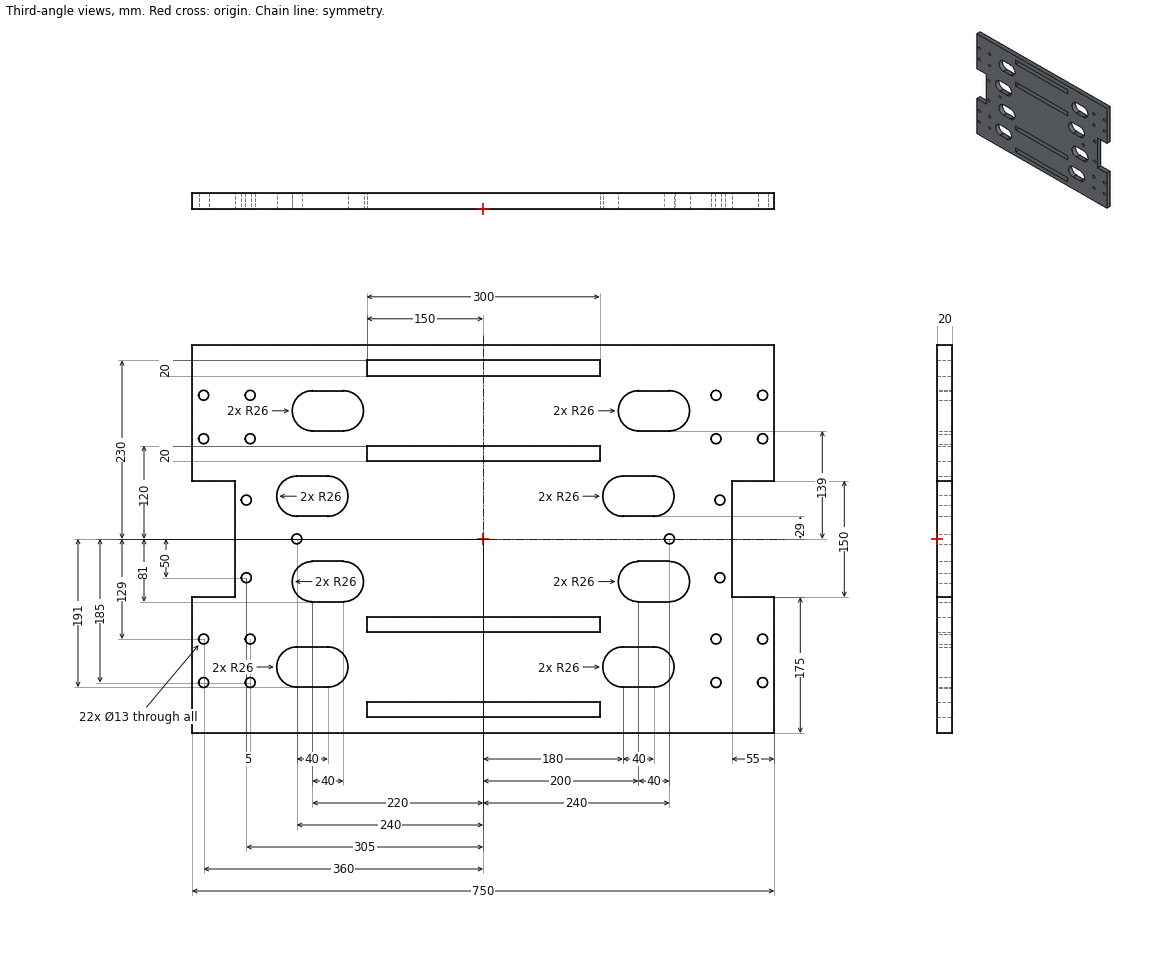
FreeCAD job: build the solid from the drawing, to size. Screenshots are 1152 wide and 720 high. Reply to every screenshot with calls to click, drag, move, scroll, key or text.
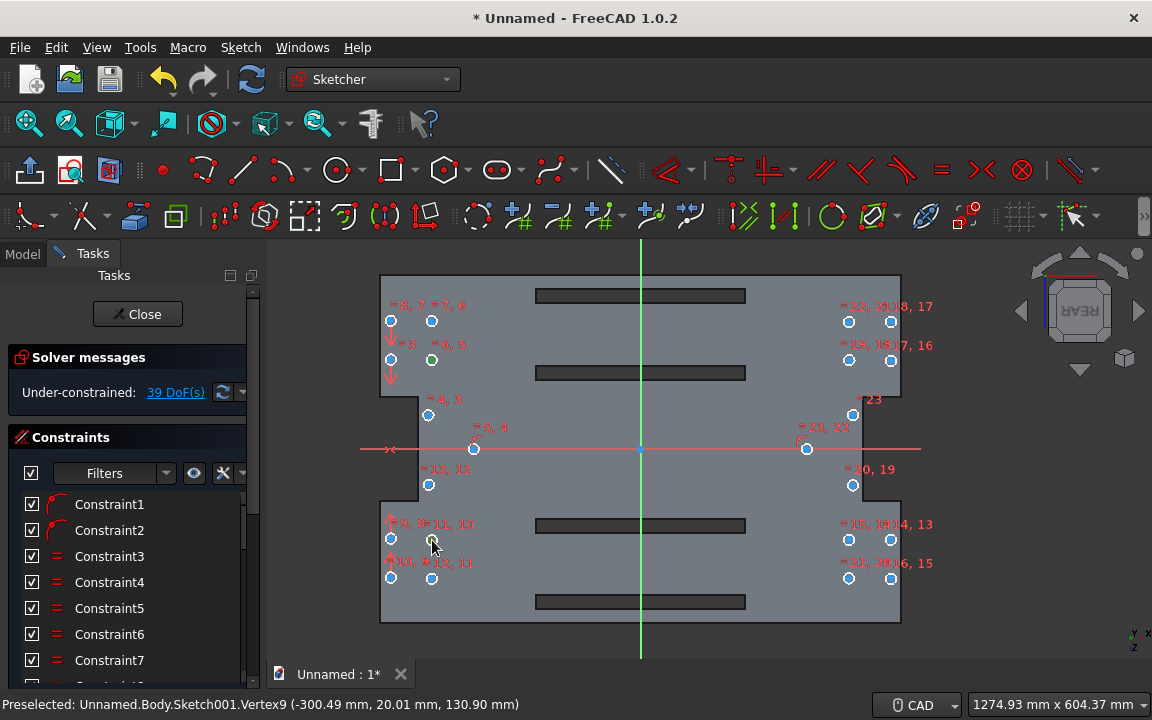
click(542, 449)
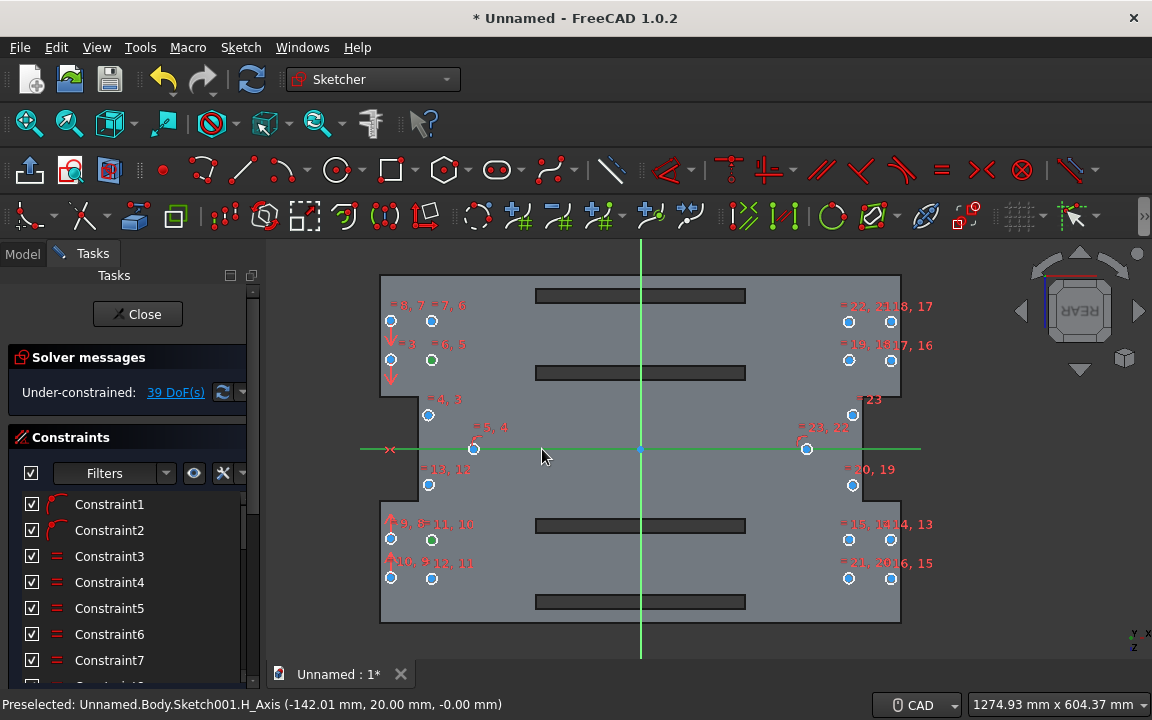
click(982, 170)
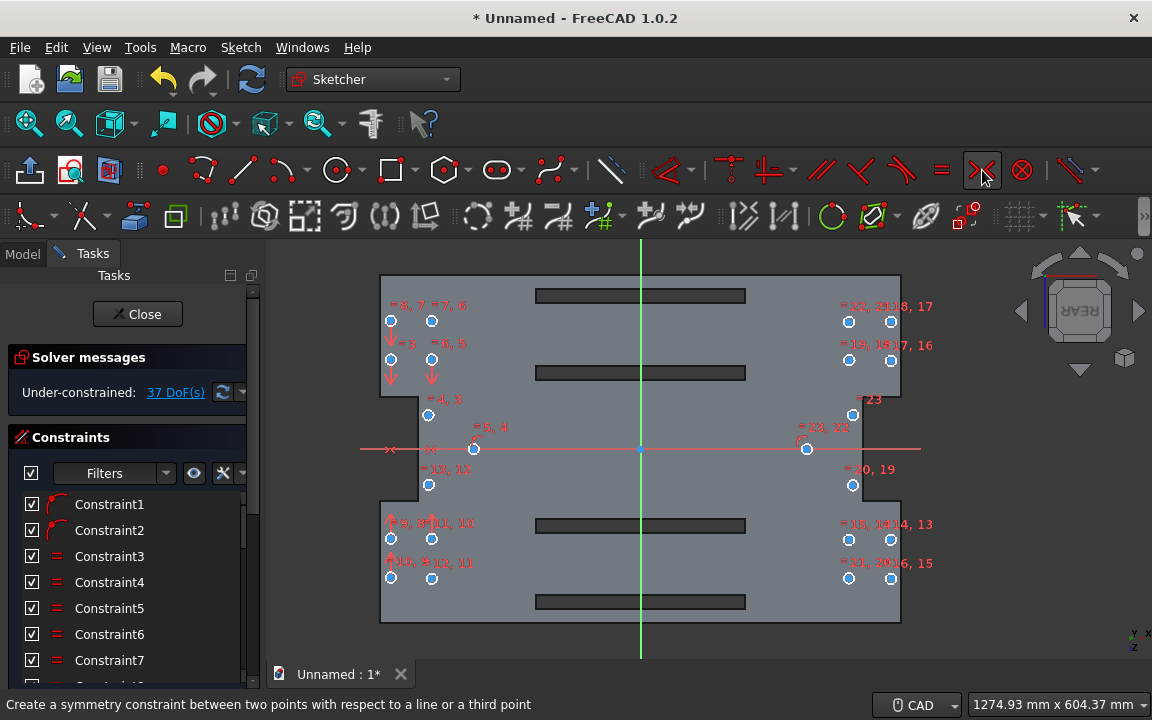
click(432, 321)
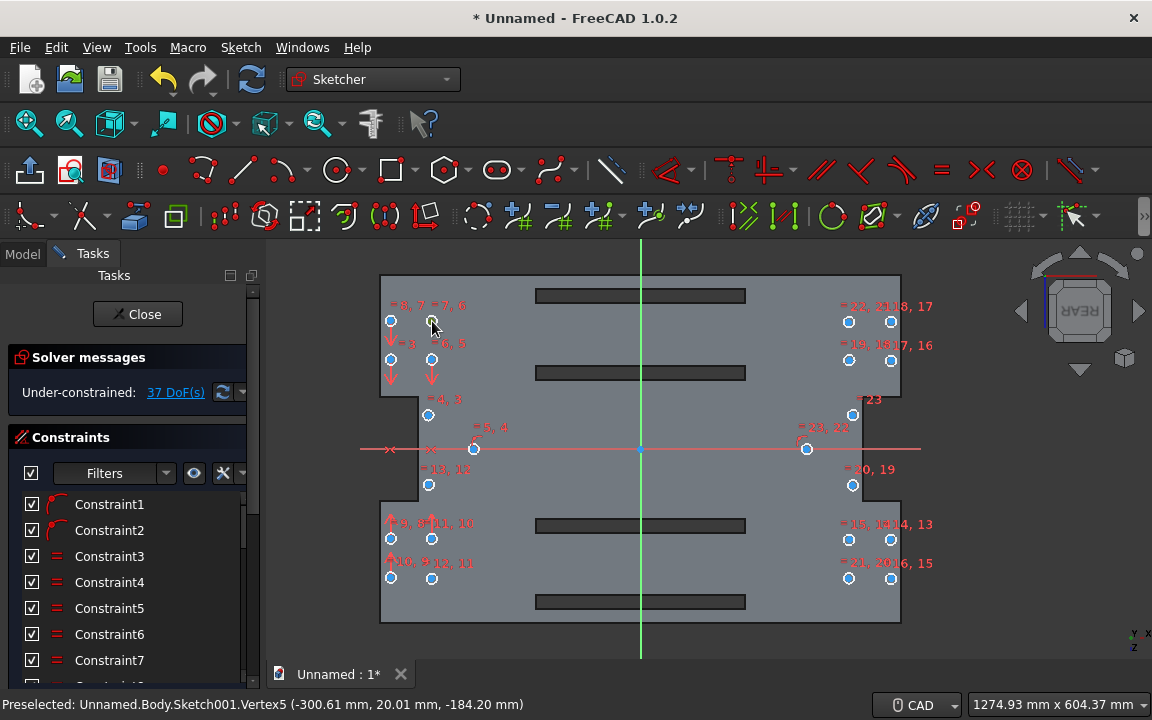
click(432, 579)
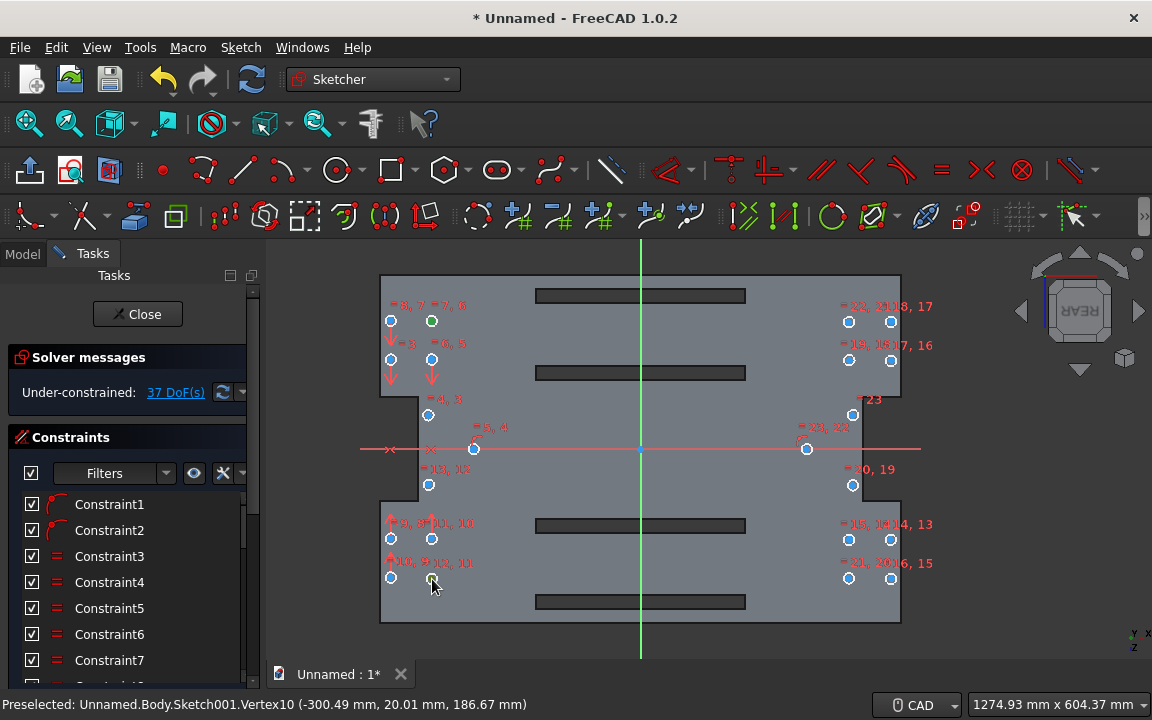
click(542, 449)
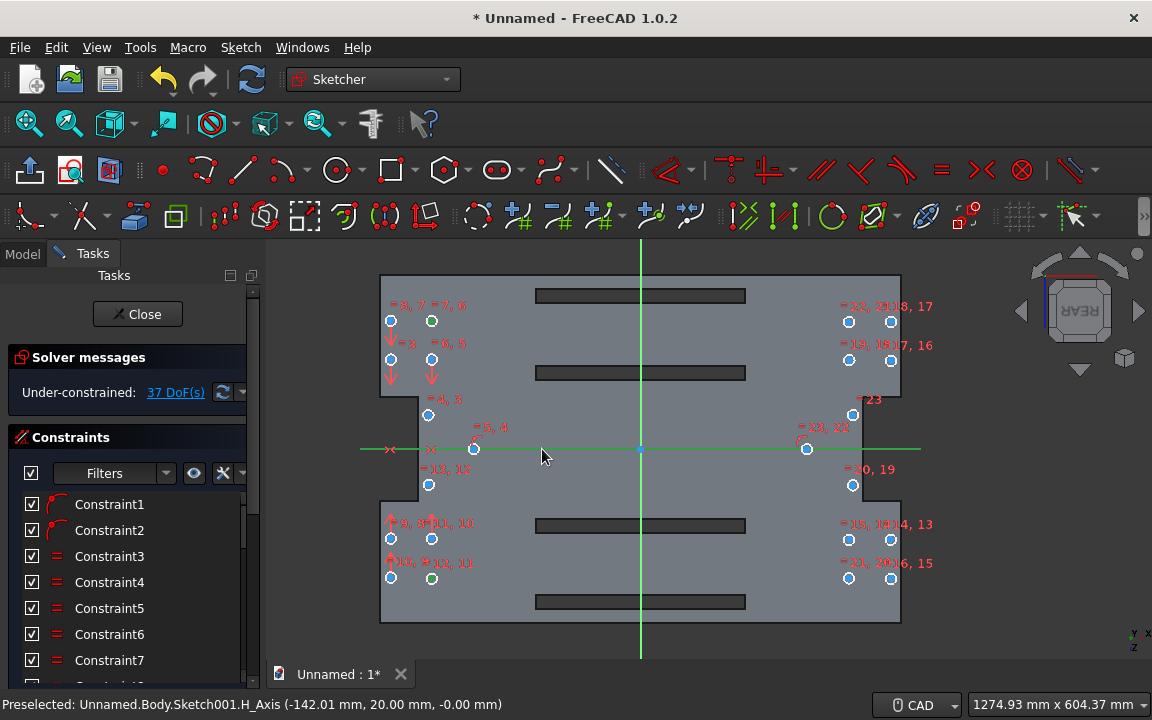
click(982, 170)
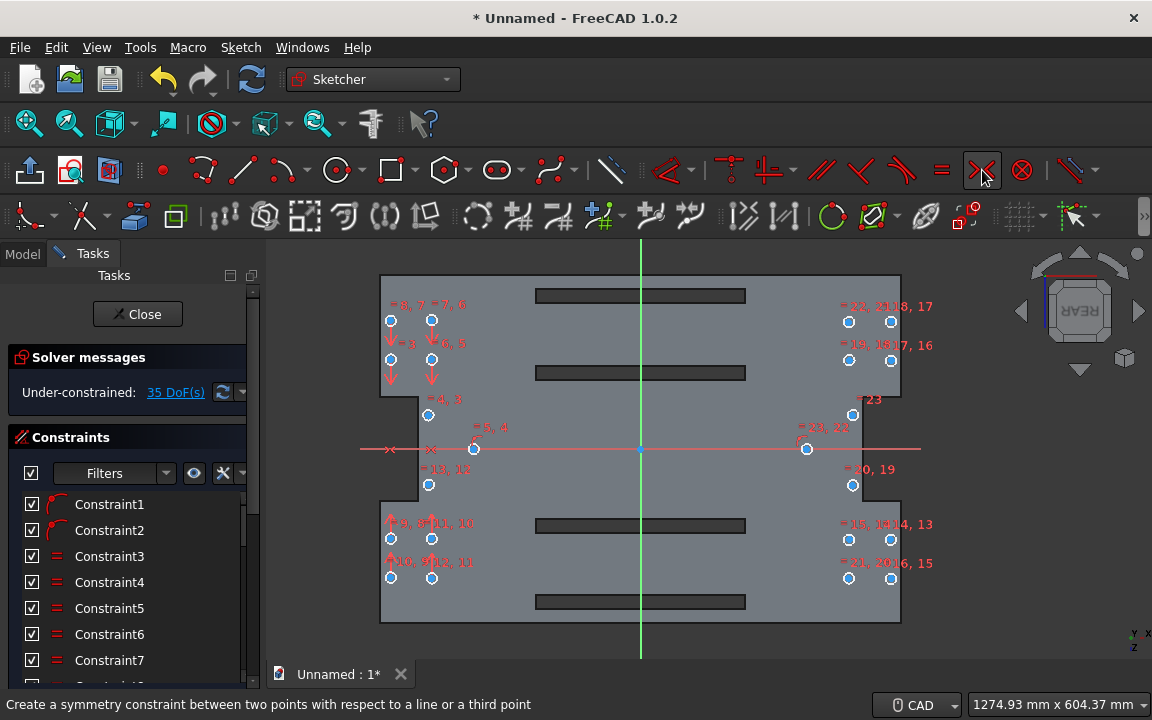
click(428, 415)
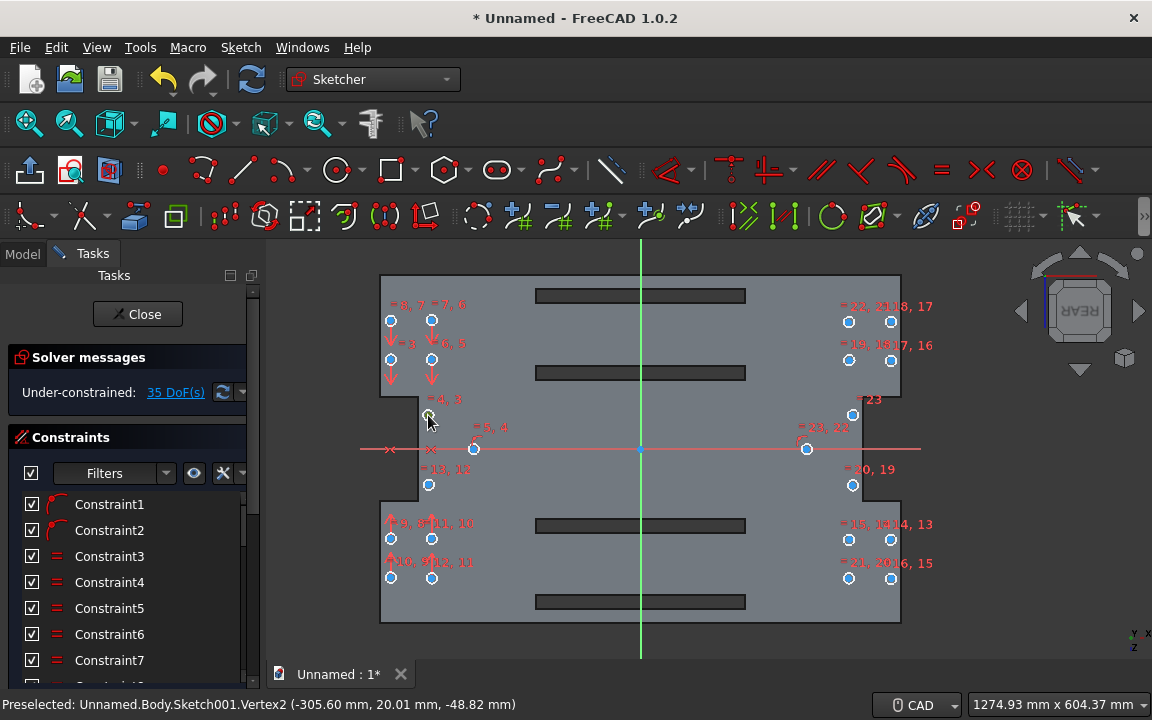
click(429, 485)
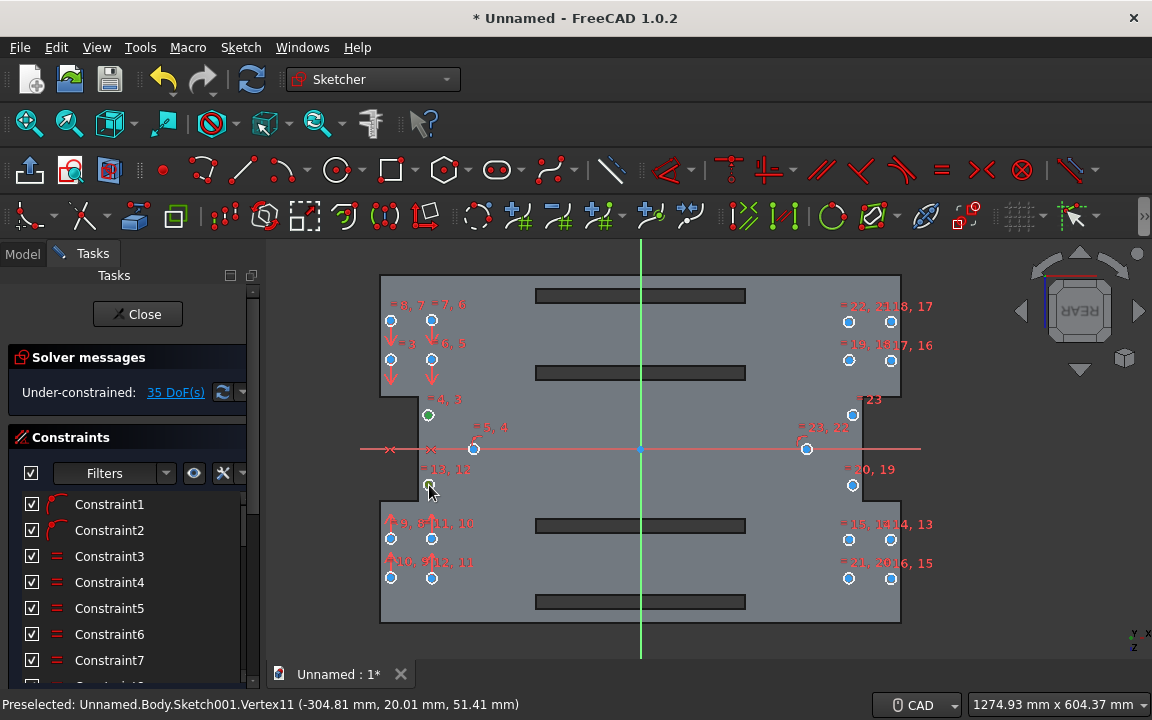
click(542, 449)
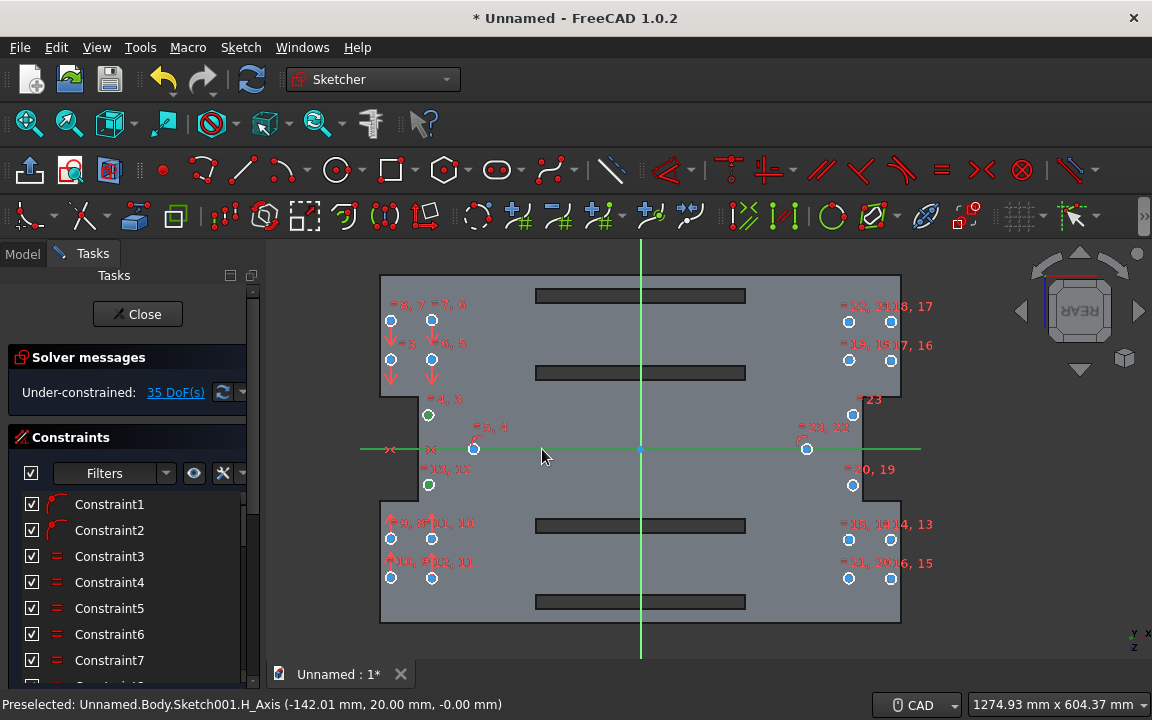
click(982, 170)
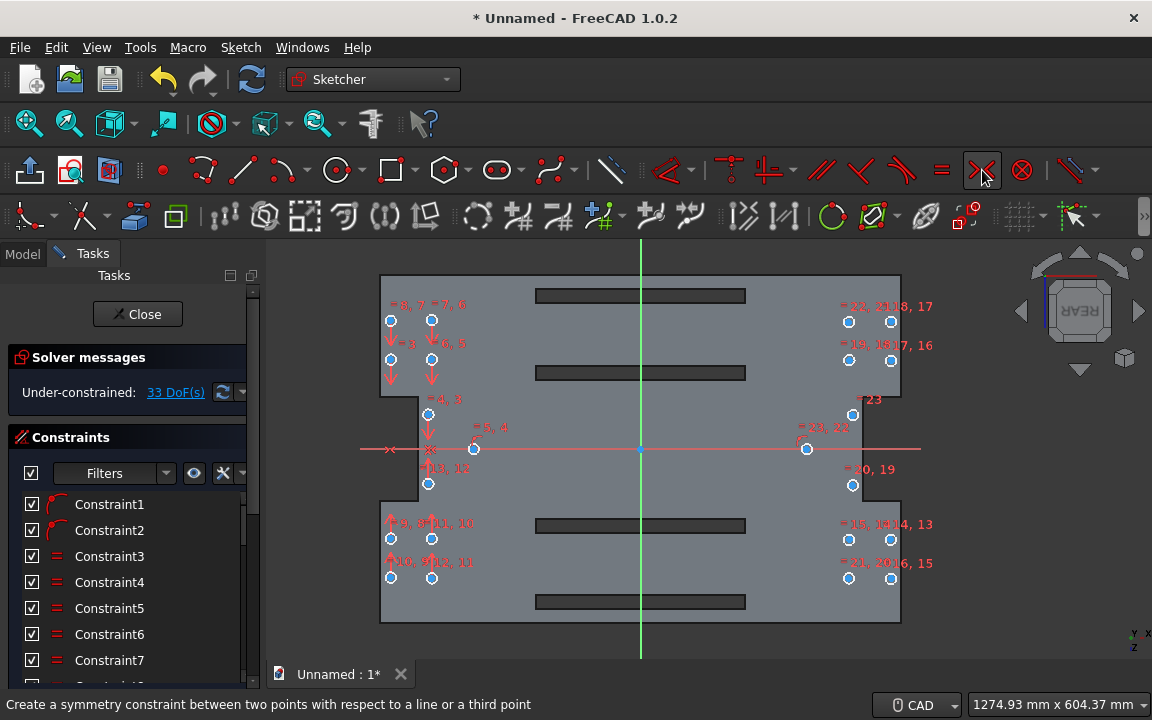
click(391, 539)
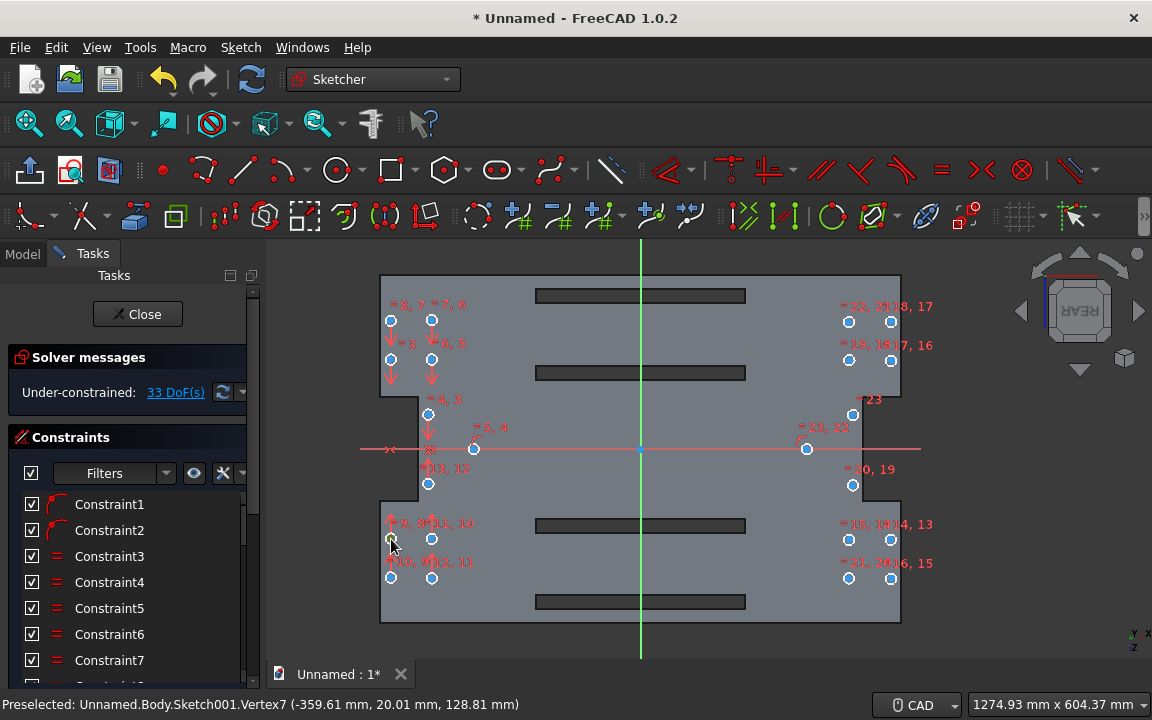
click(891, 540)